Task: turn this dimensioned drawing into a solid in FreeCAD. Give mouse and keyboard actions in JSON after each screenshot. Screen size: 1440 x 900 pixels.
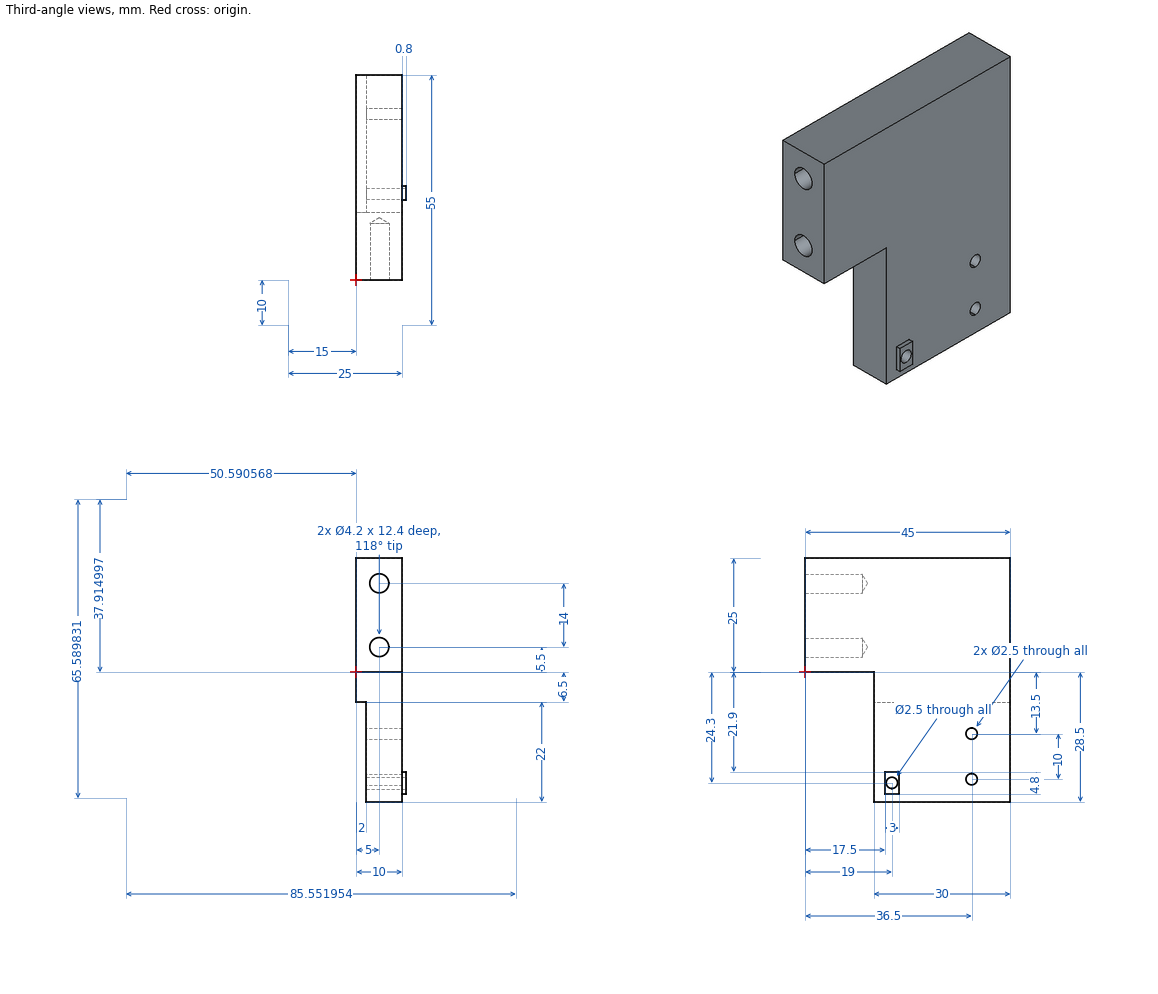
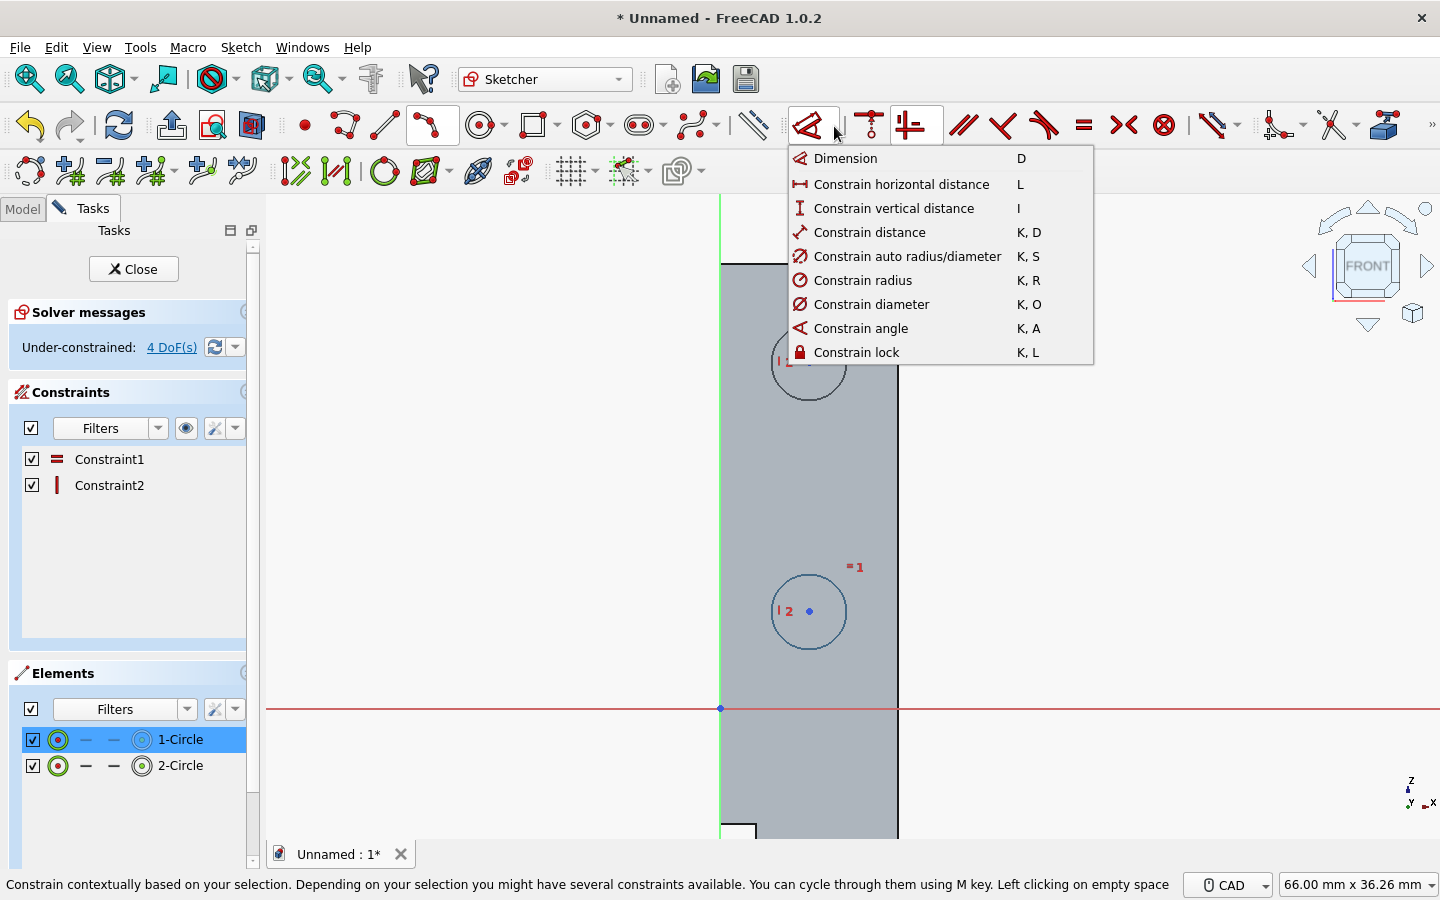
{"action": "left_click", "coordinate": [941, 304]}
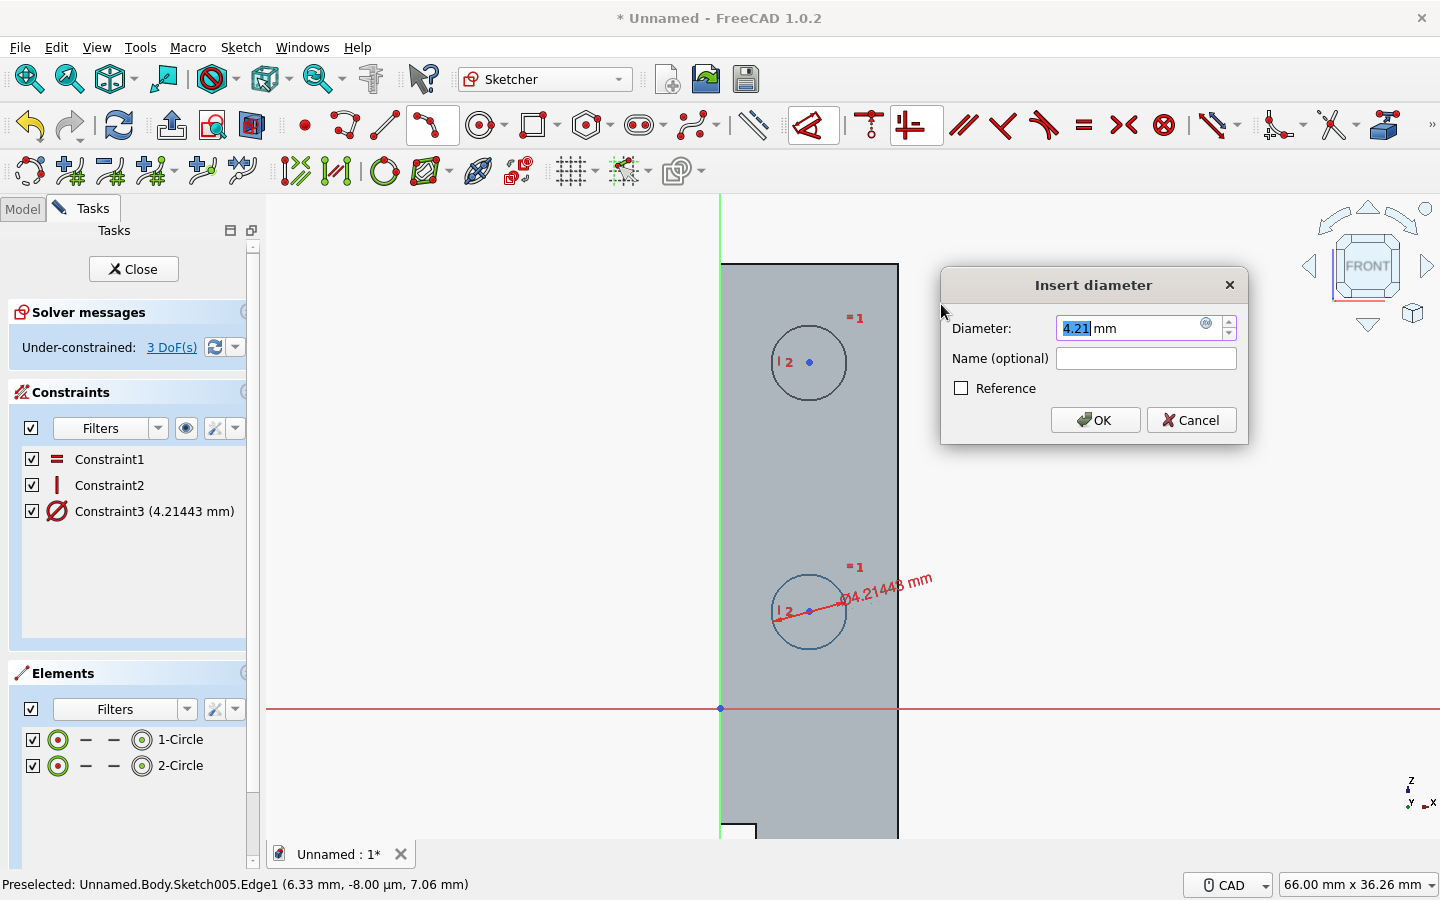
{"action": "type", "text": "4.2"}
{"action": "key", "text": "Return"}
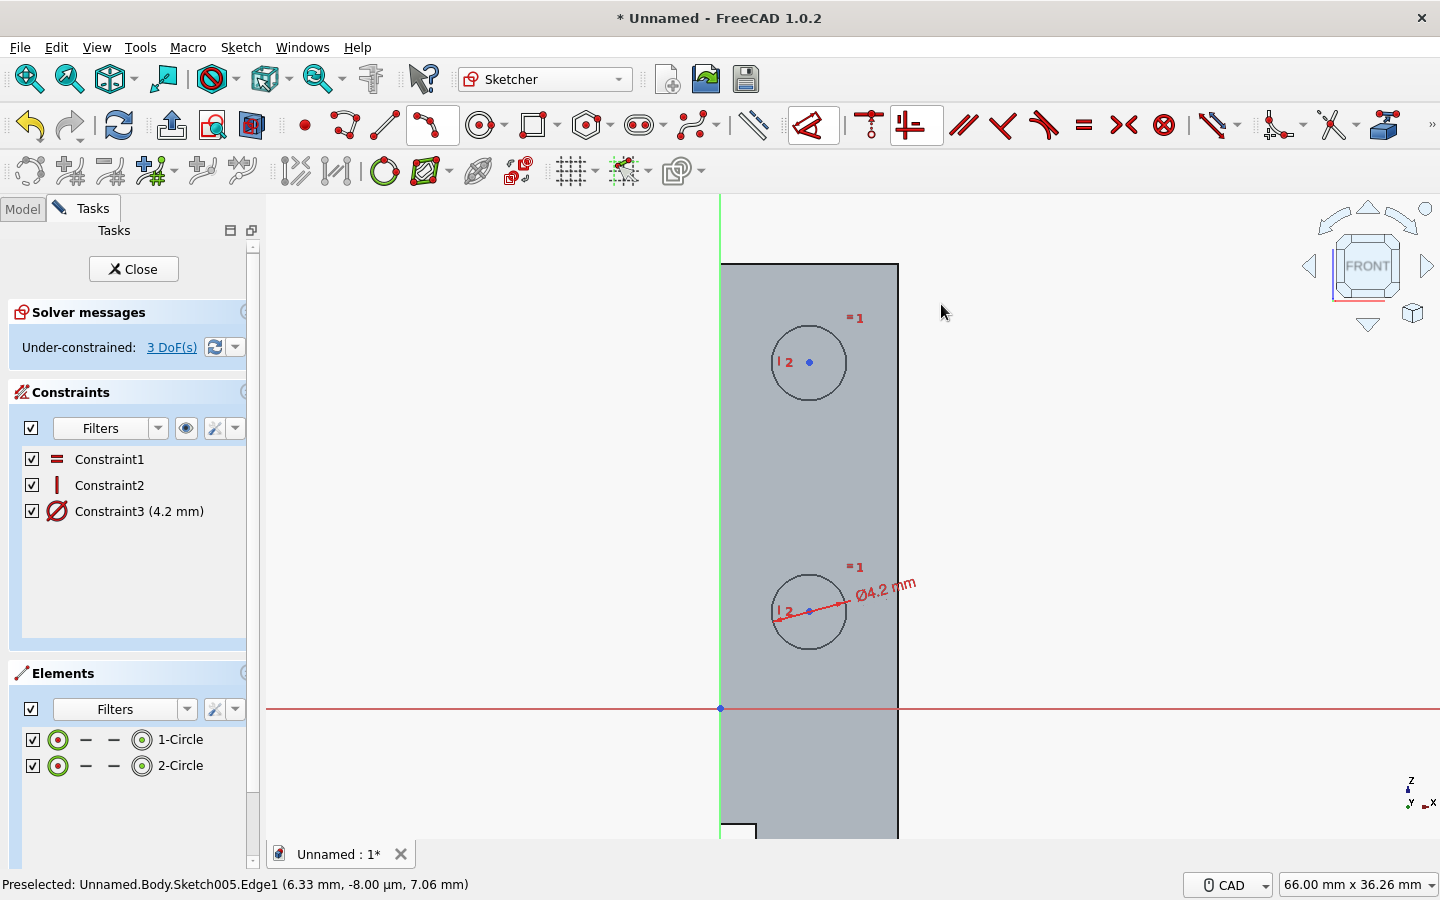
{"action": "left_click", "coordinate": [809, 612]}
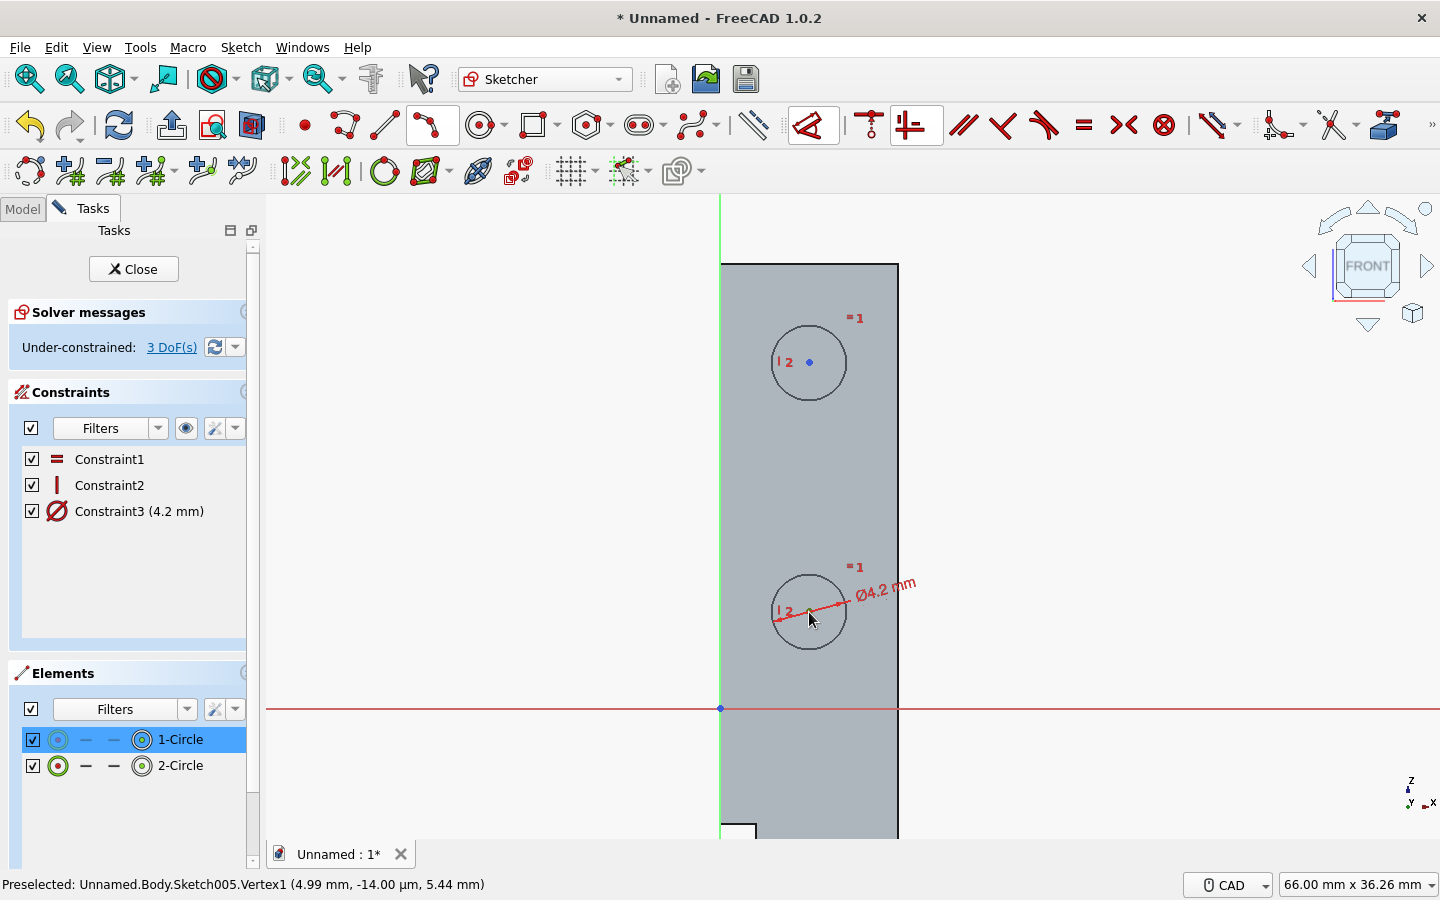
{"action": "left_click", "coordinate": [834, 126]}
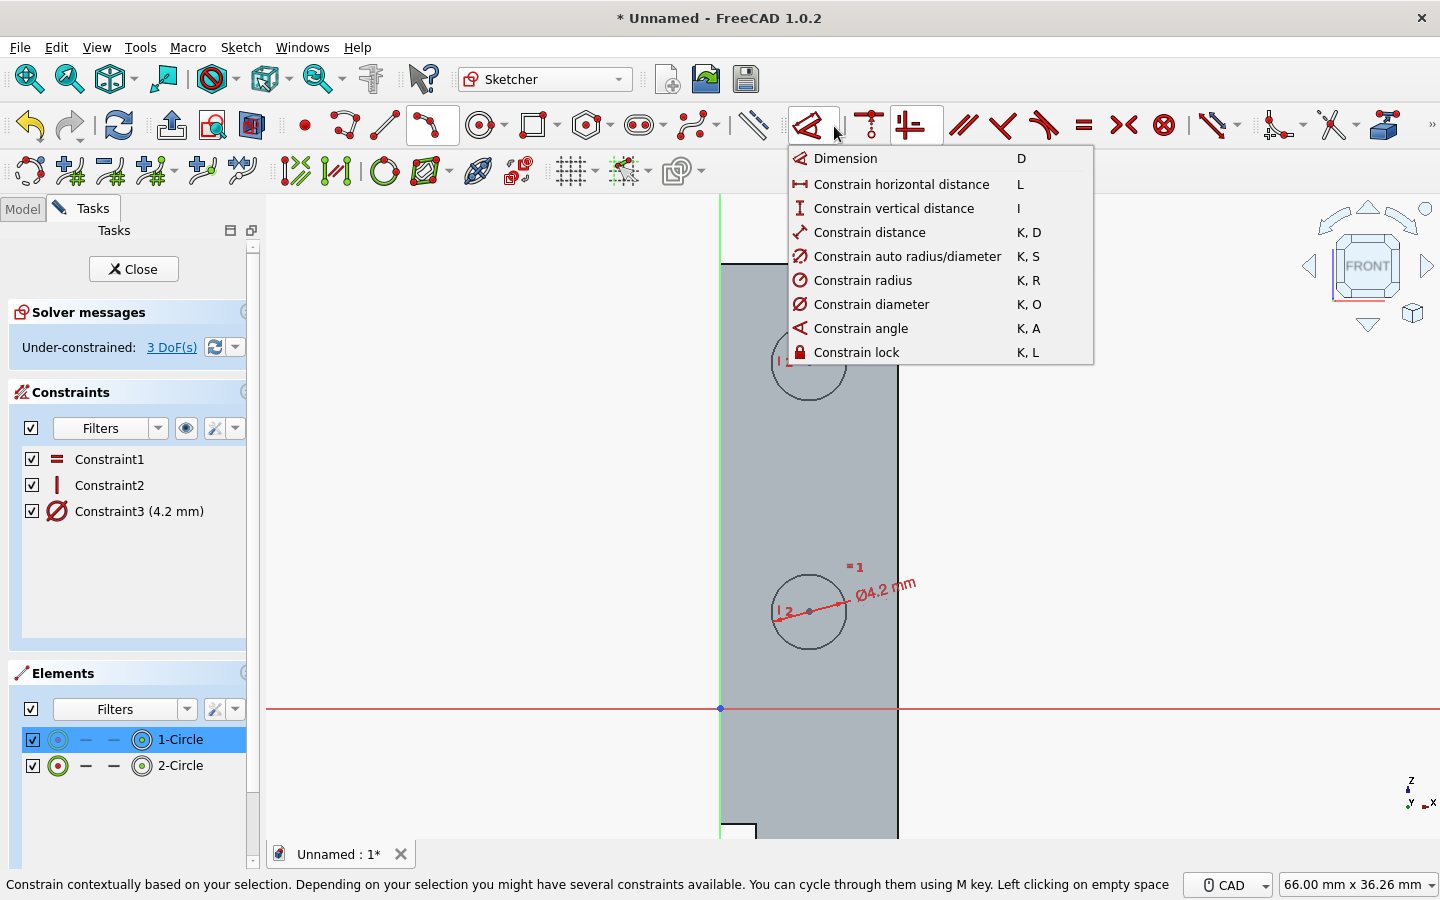
{"action": "left_click", "coordinate": [941, 184]}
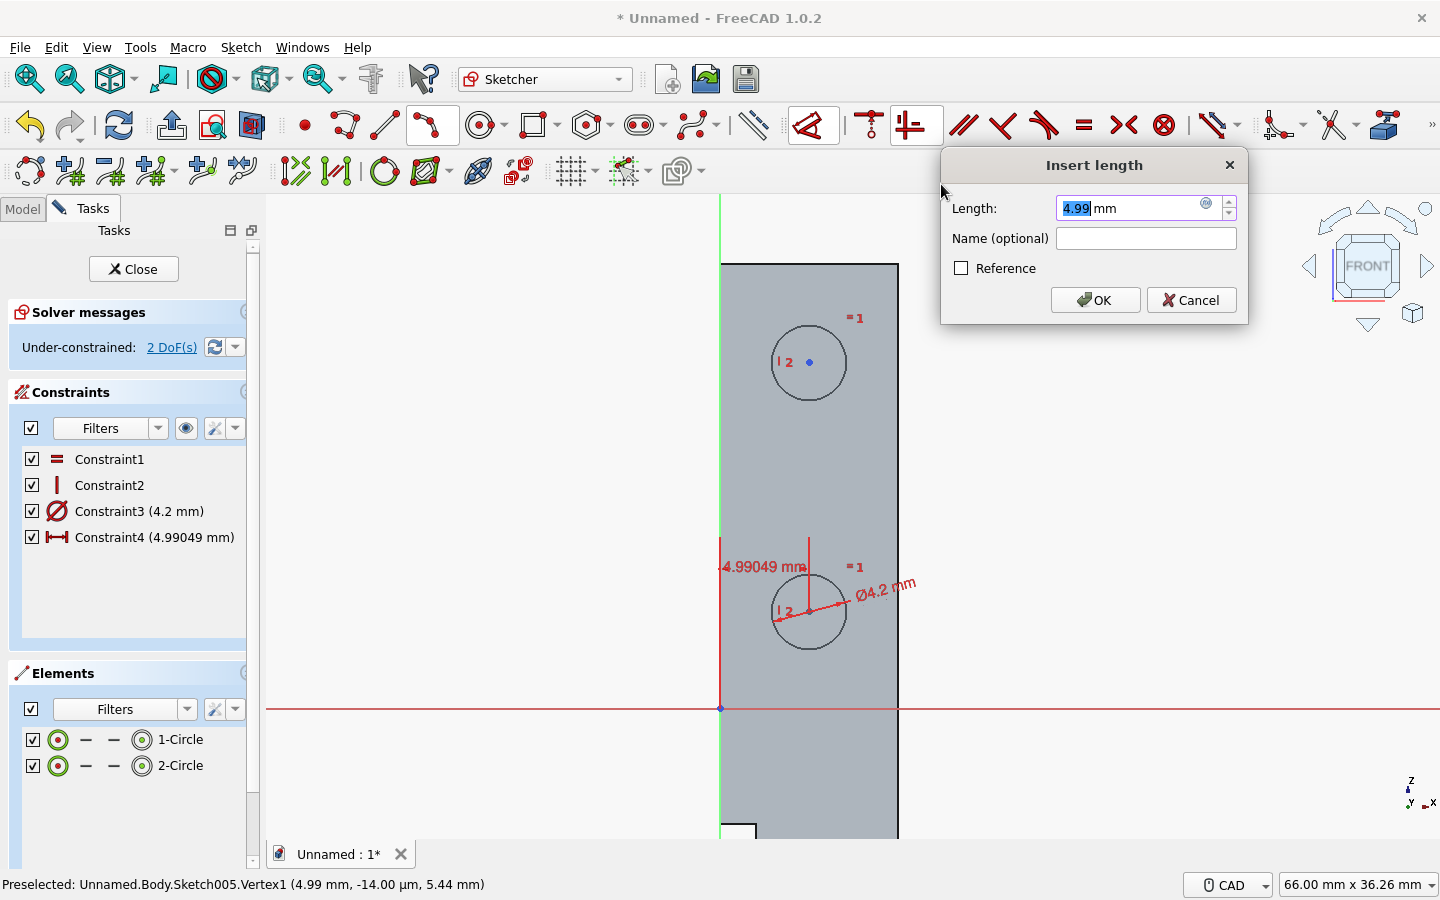
{"action": "type", "text": "5"}
{"action": "key", "text": "Return"}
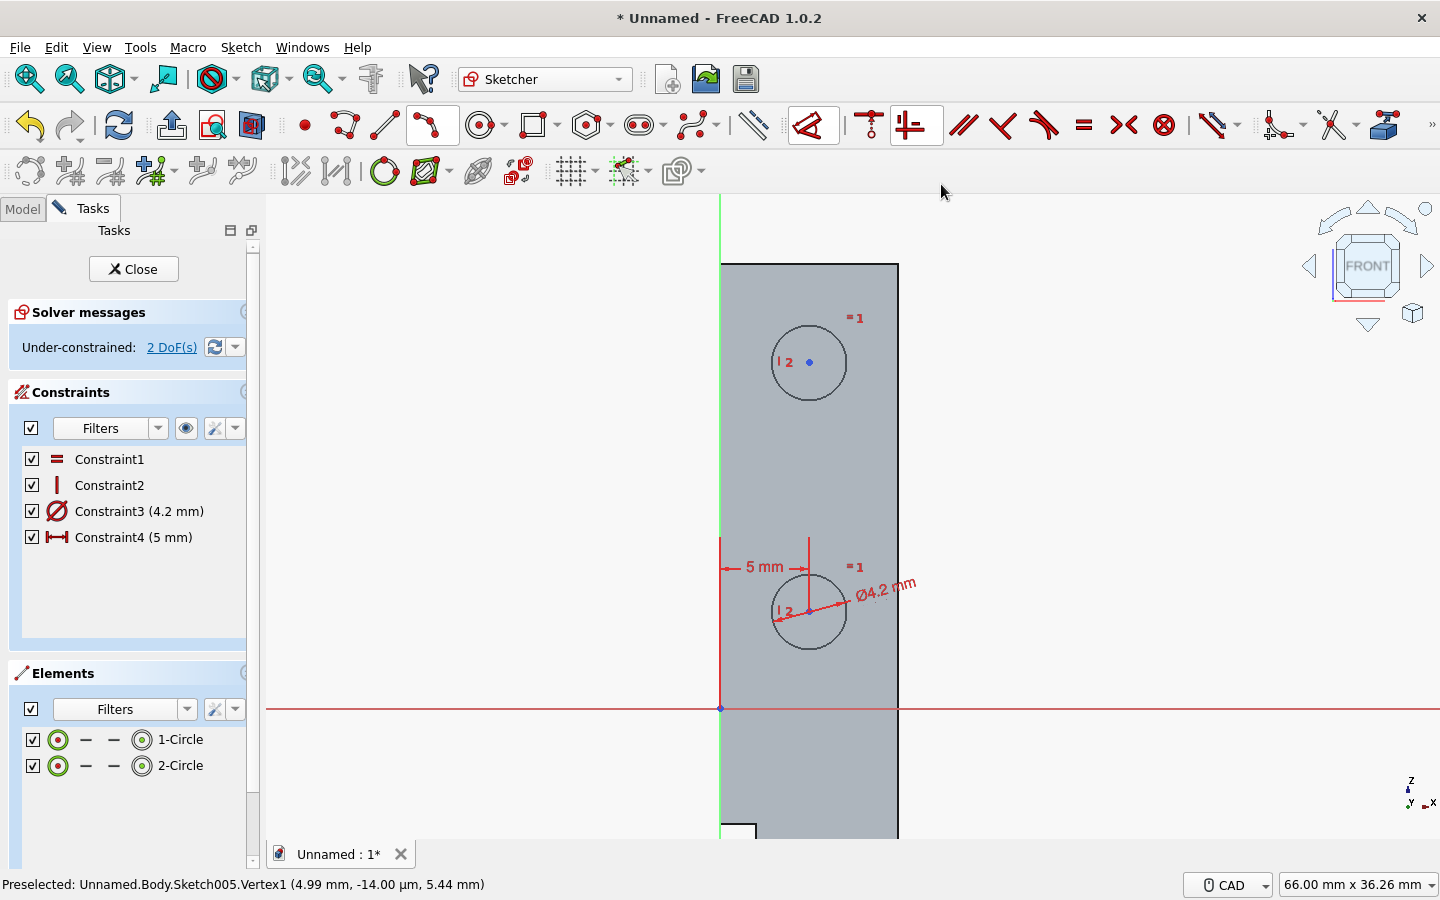
{"action": "left_click", "coordinate": [809, 612]}